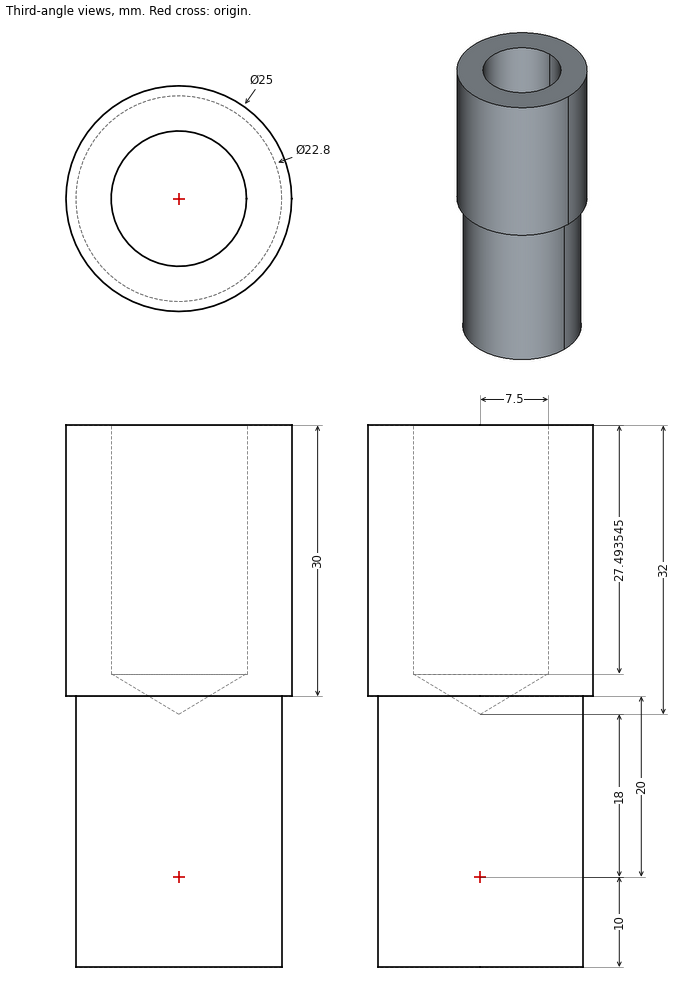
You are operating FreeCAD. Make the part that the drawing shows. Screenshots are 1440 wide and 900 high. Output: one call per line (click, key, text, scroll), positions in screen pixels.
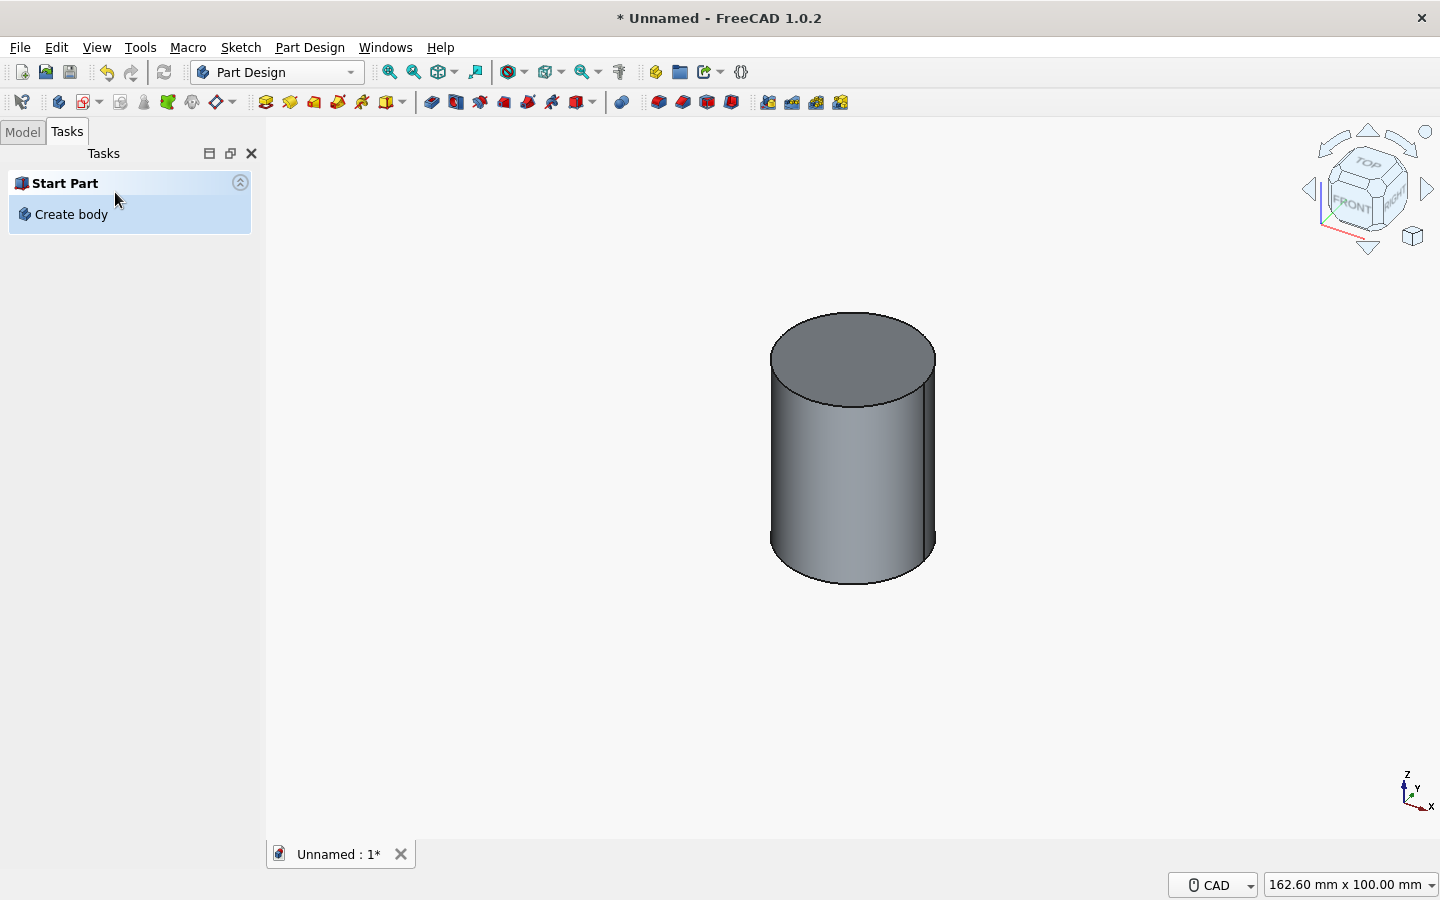
click(390, 72)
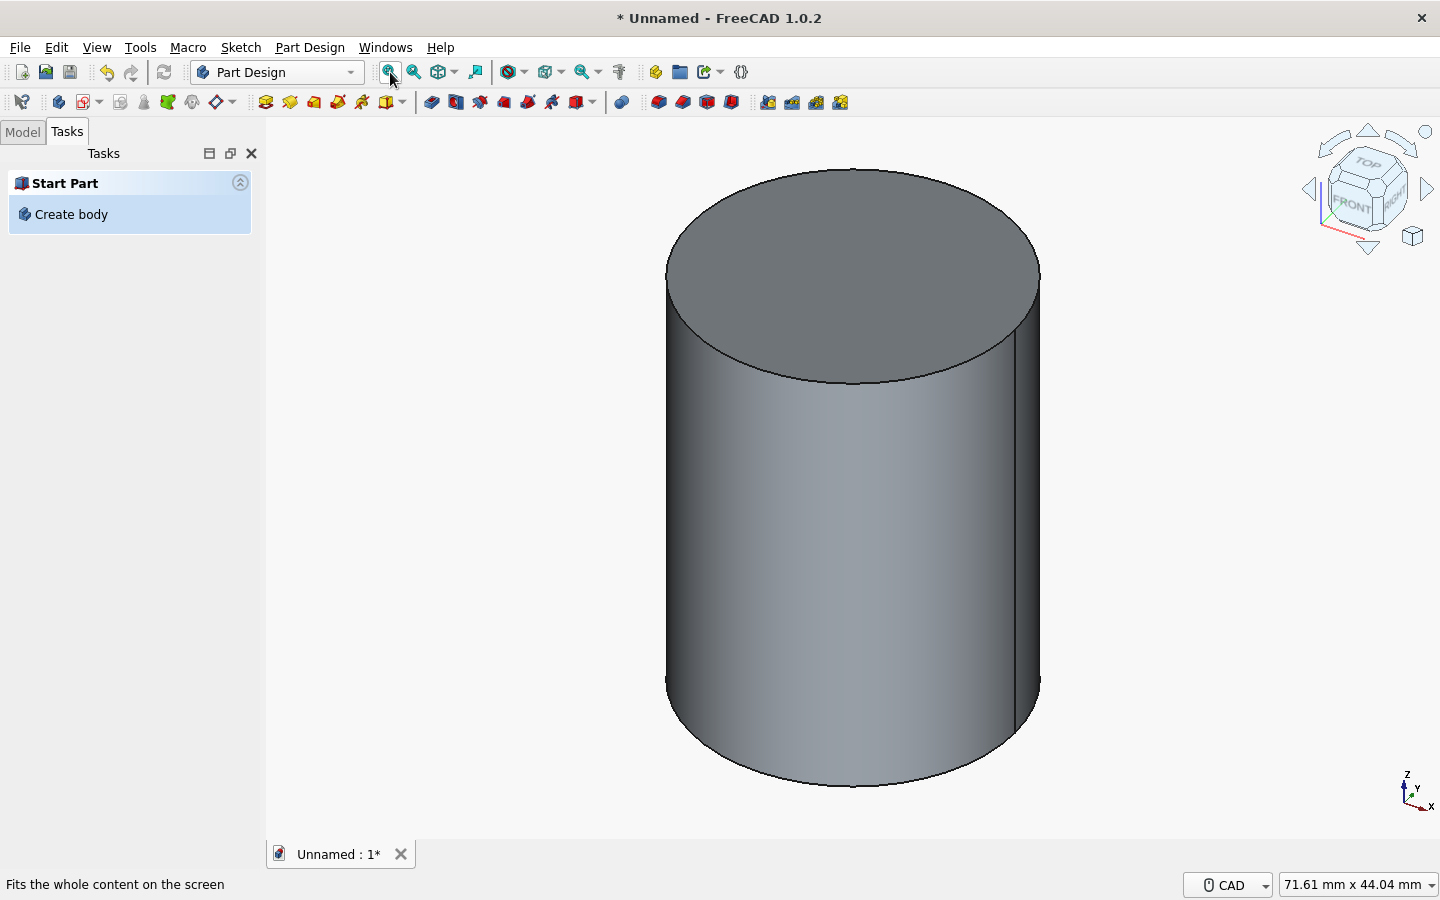
click(853, 276)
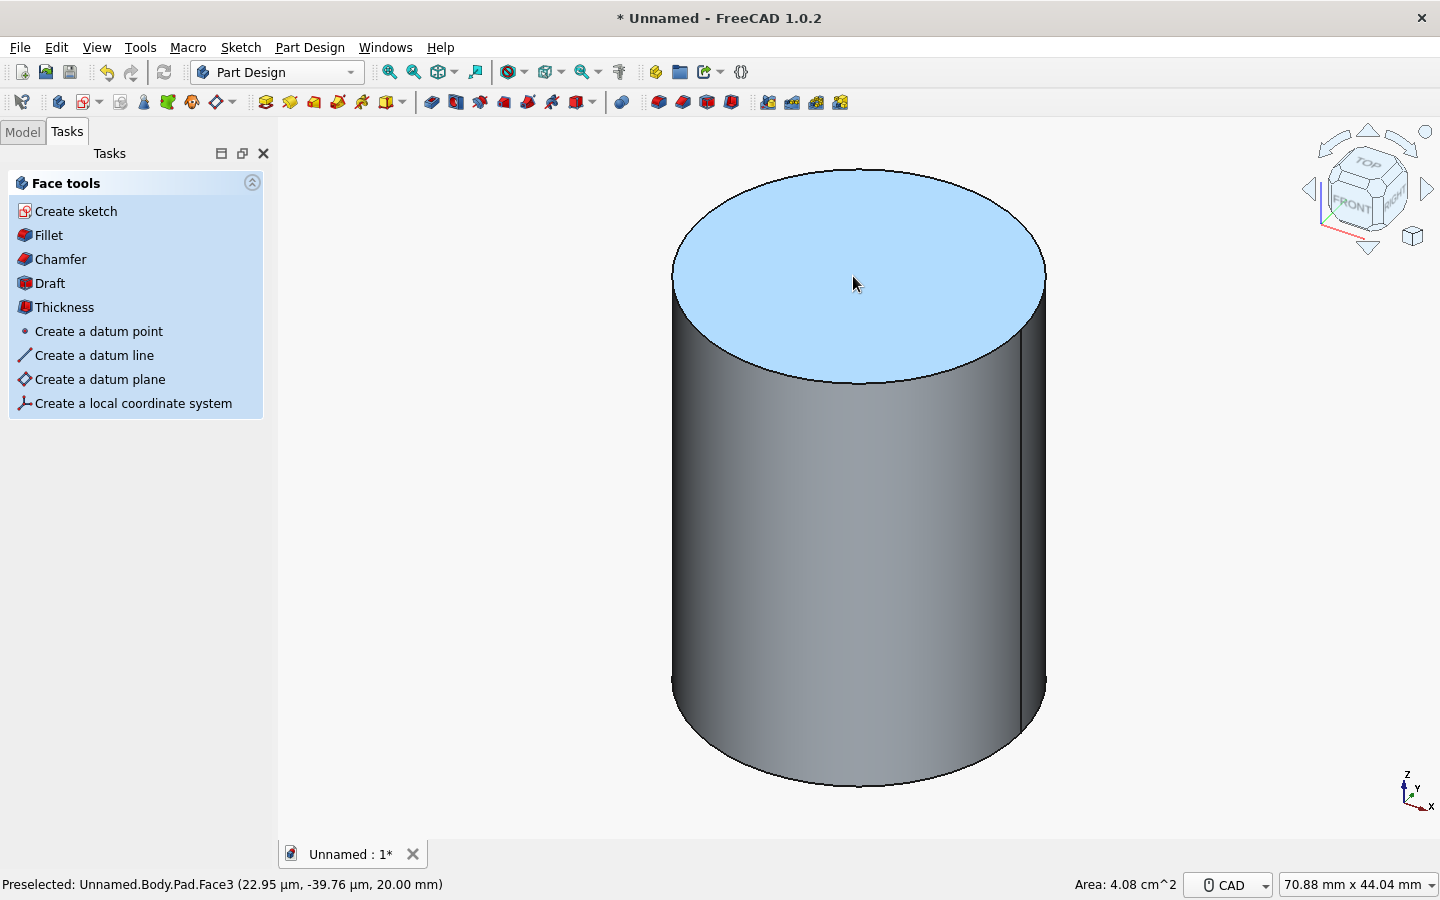
click(84, 102)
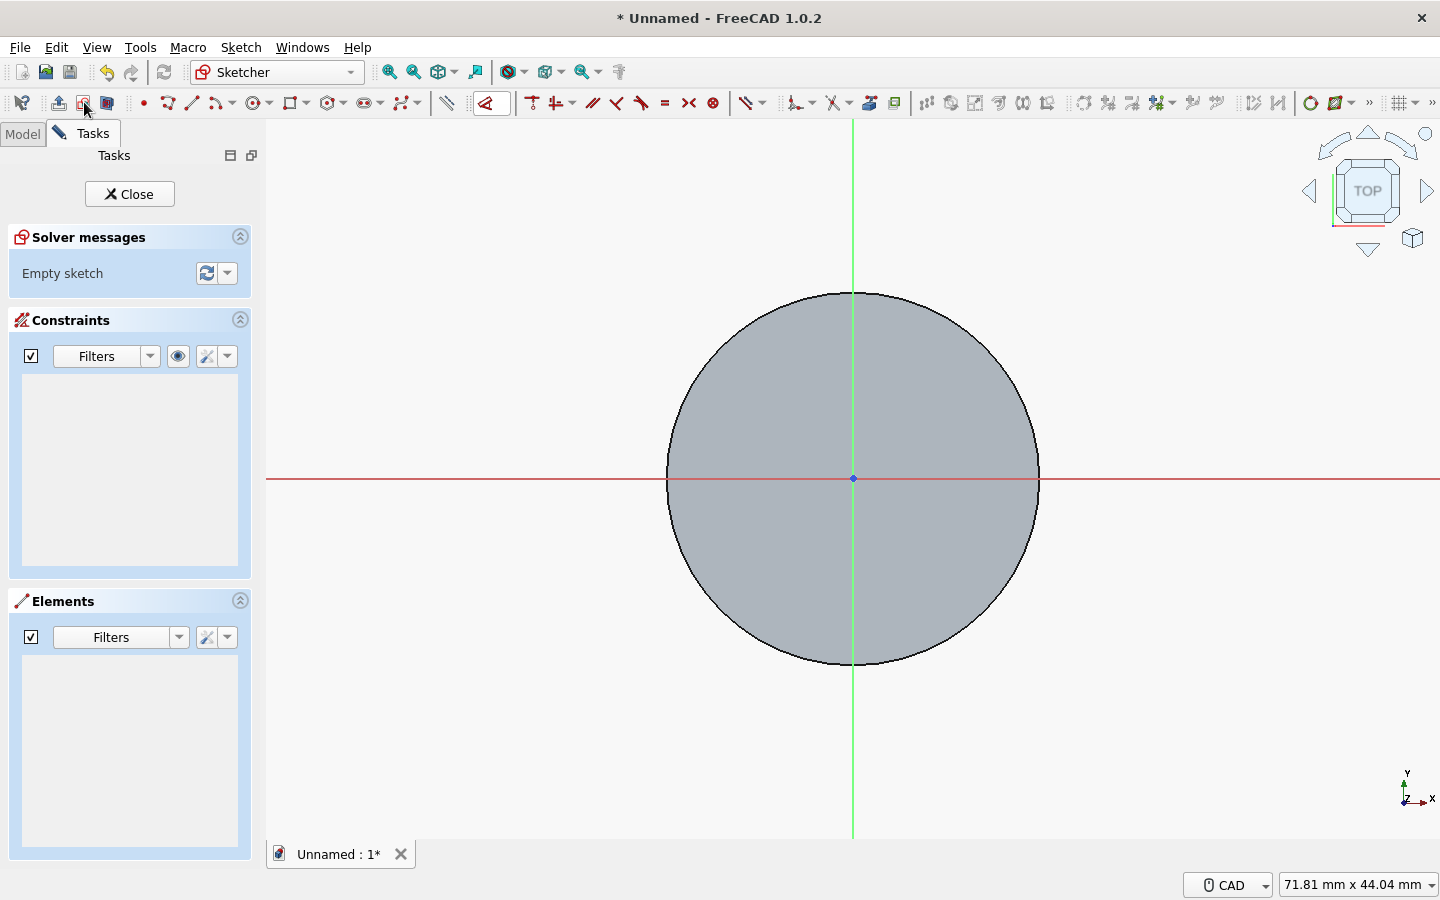
key(g)
key(c)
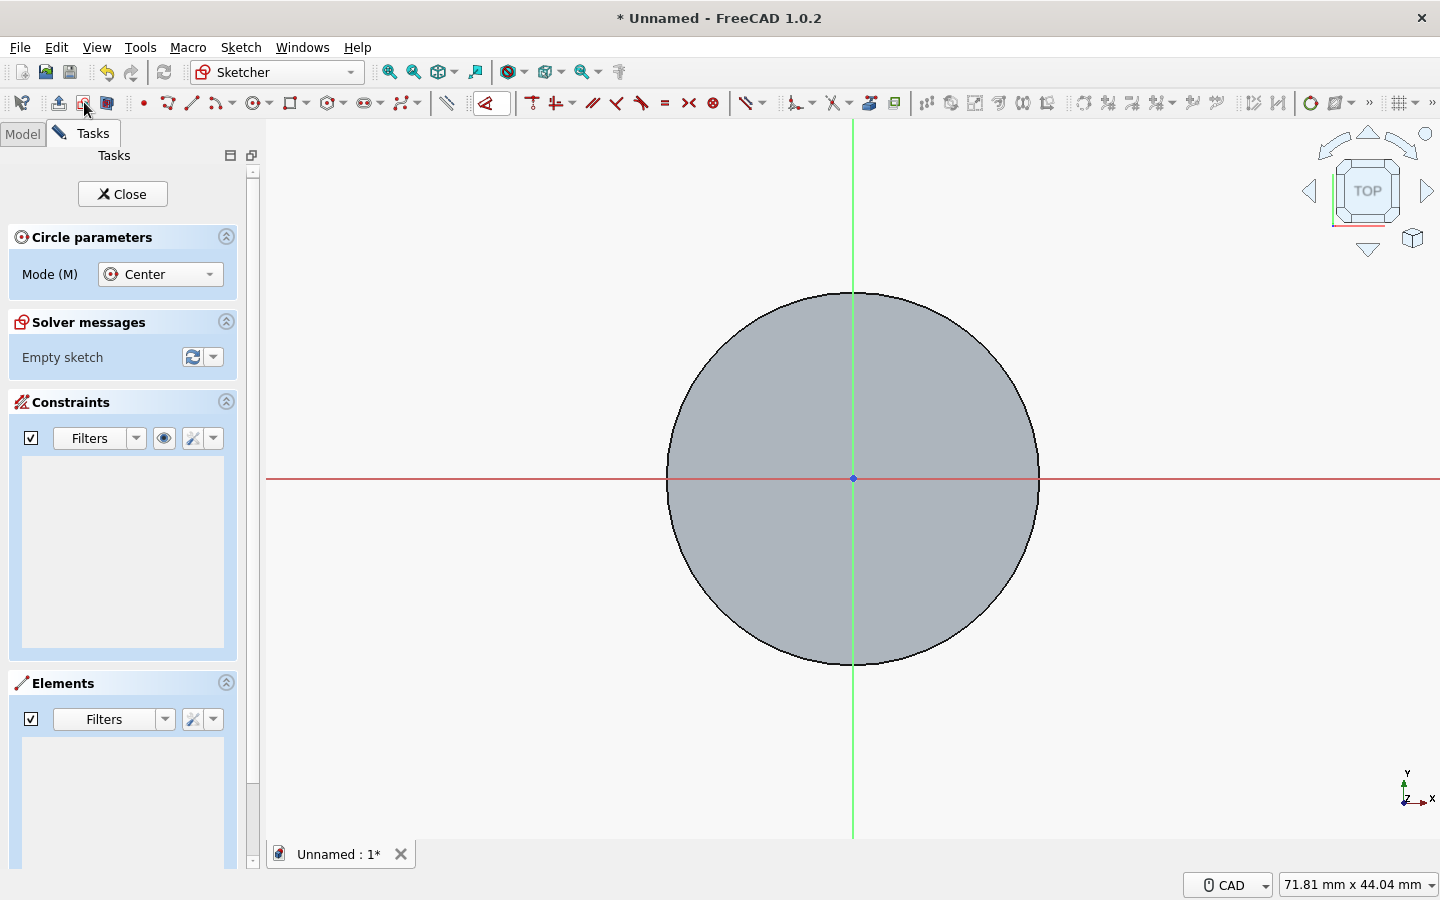
click(853, 479)
move(997, 335)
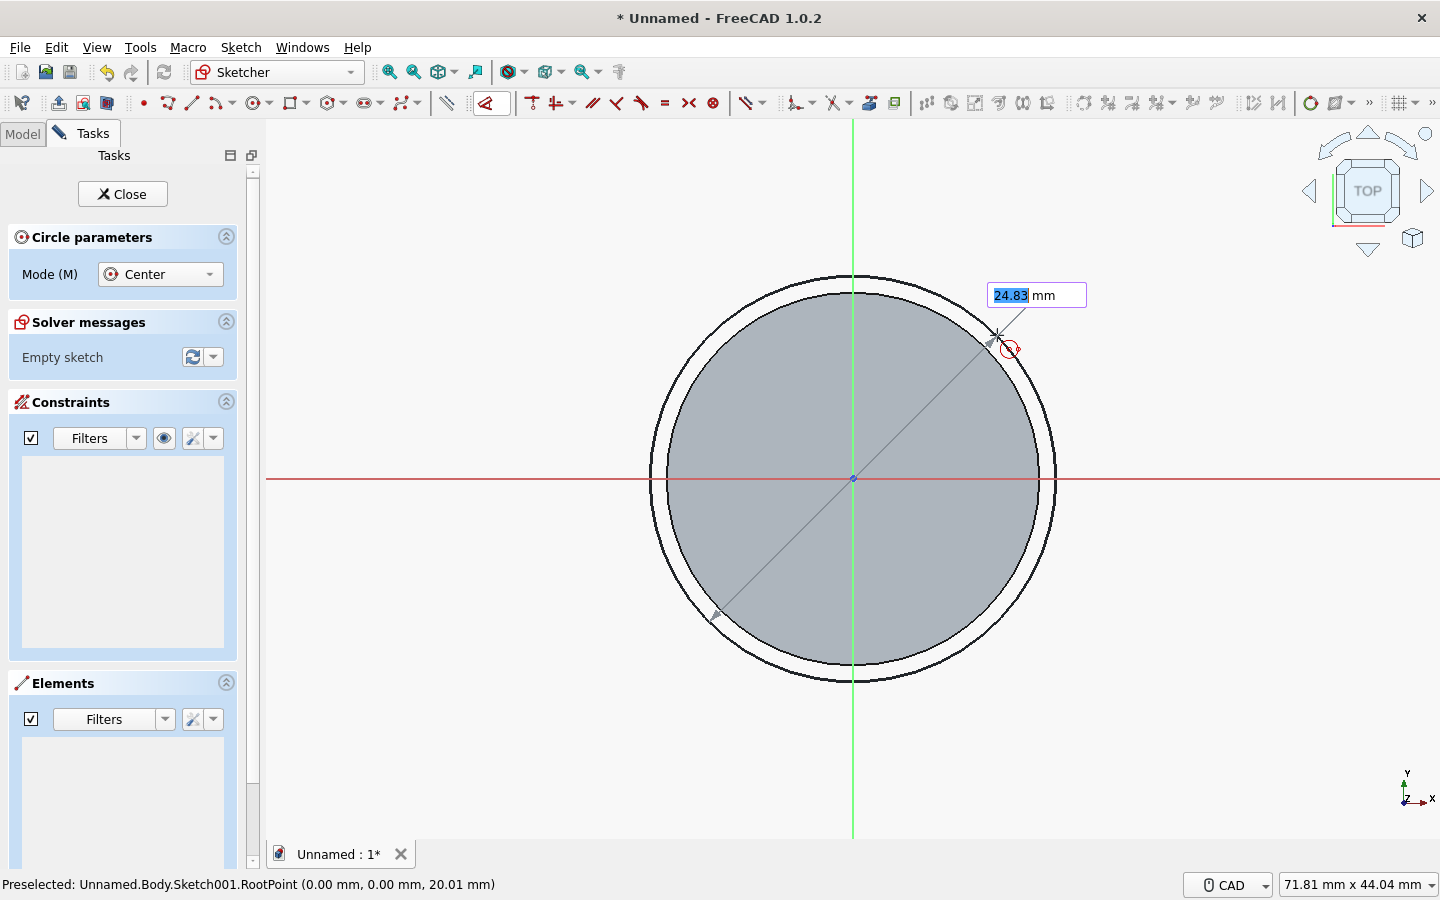
text(25)
key(Return)
key(Escape)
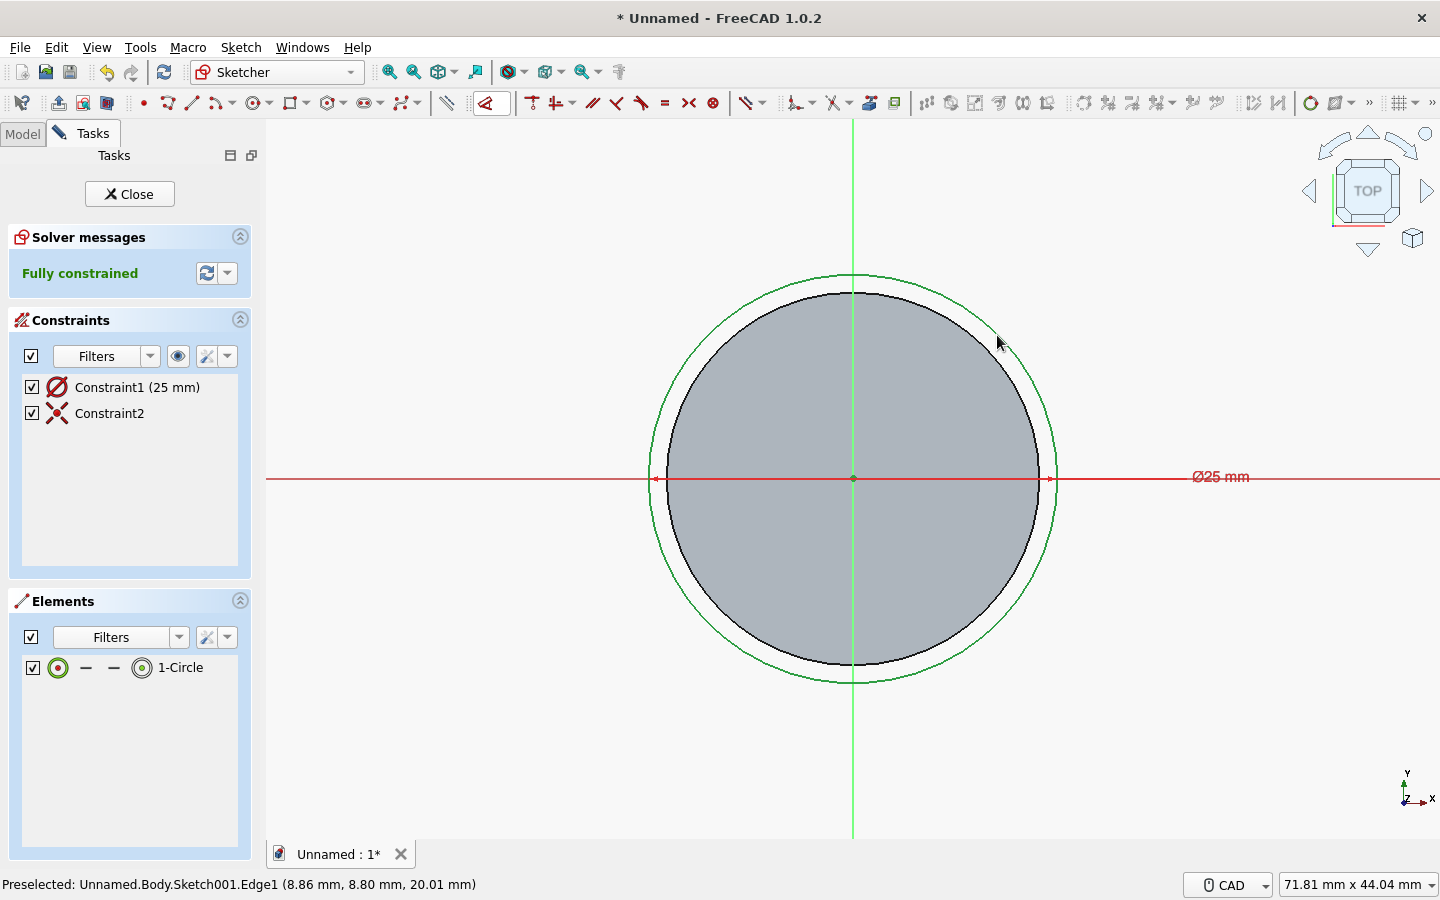
click(130, 194)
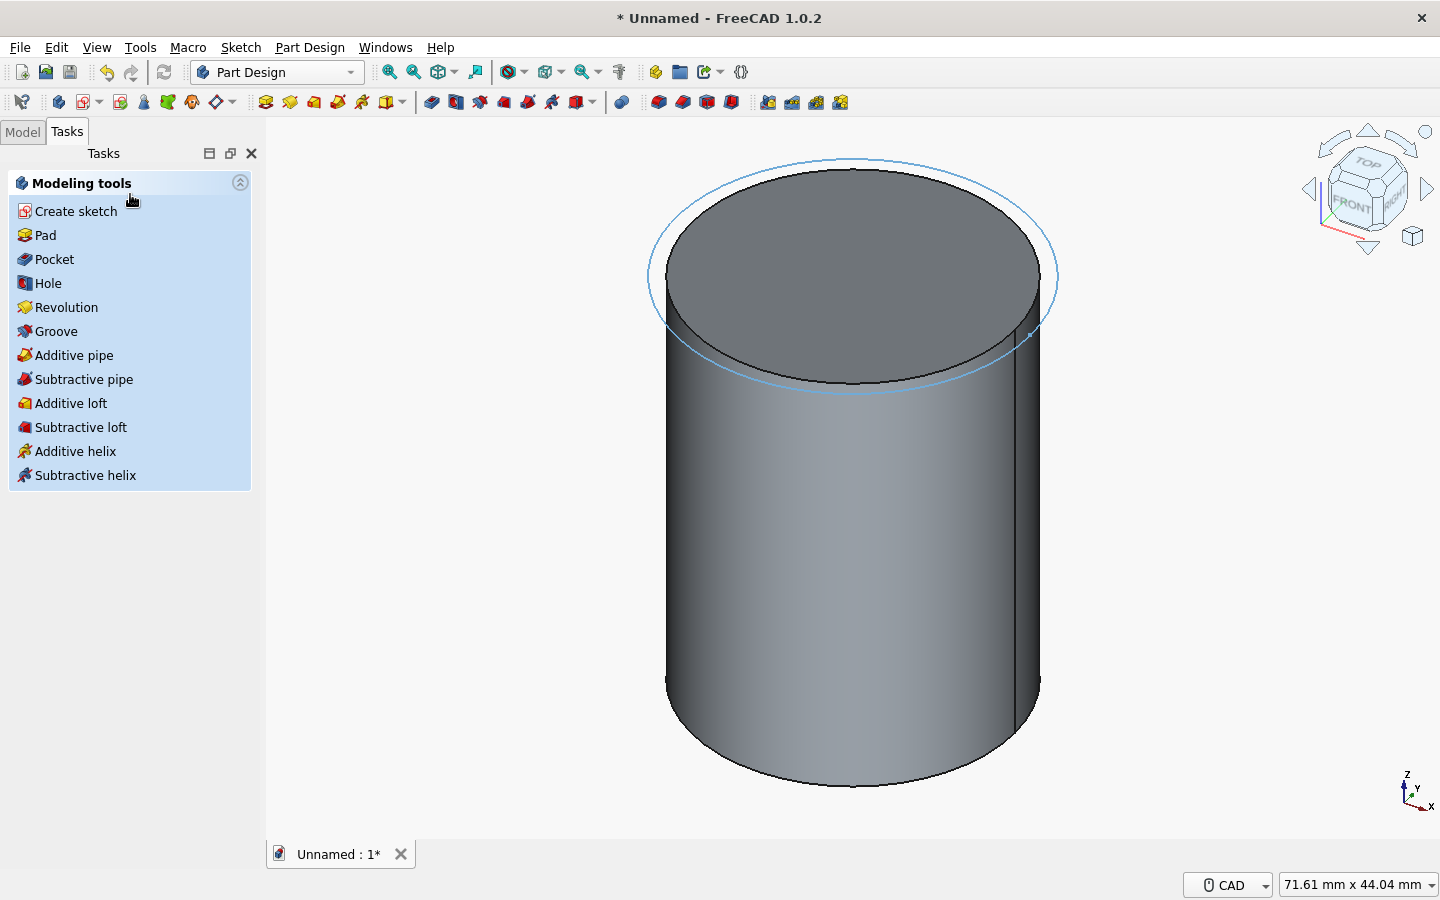
click(266, 102)